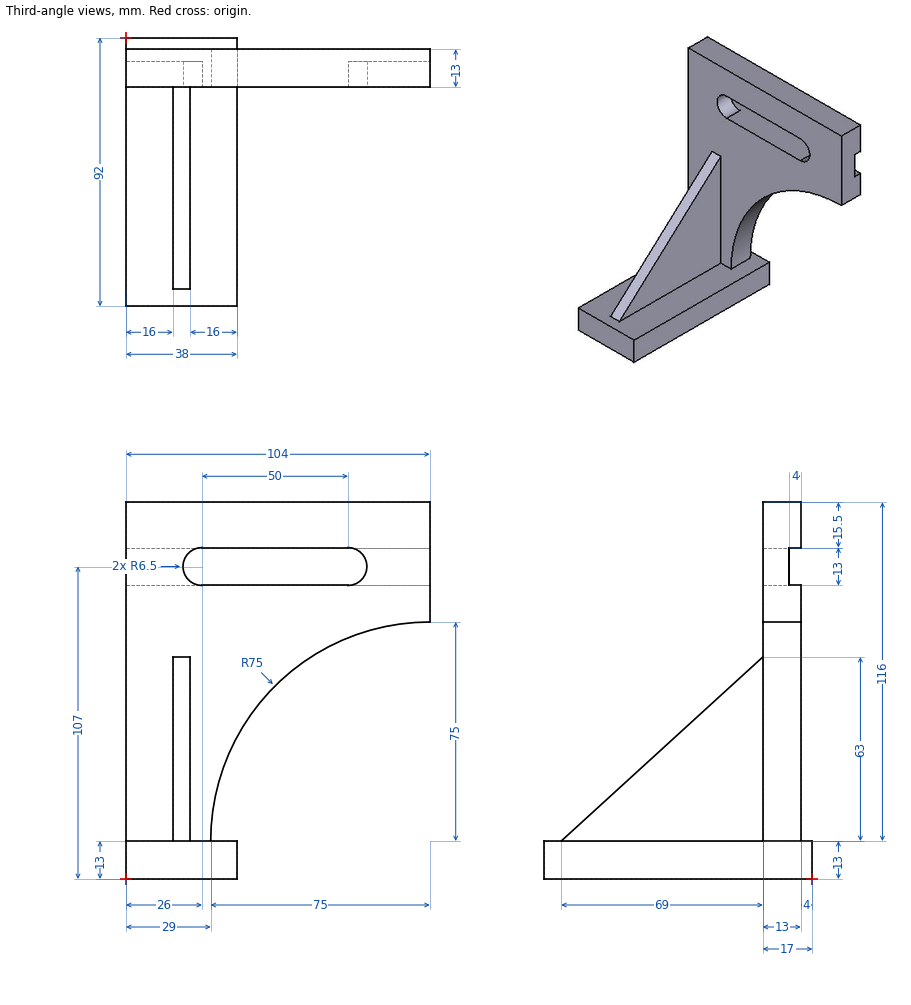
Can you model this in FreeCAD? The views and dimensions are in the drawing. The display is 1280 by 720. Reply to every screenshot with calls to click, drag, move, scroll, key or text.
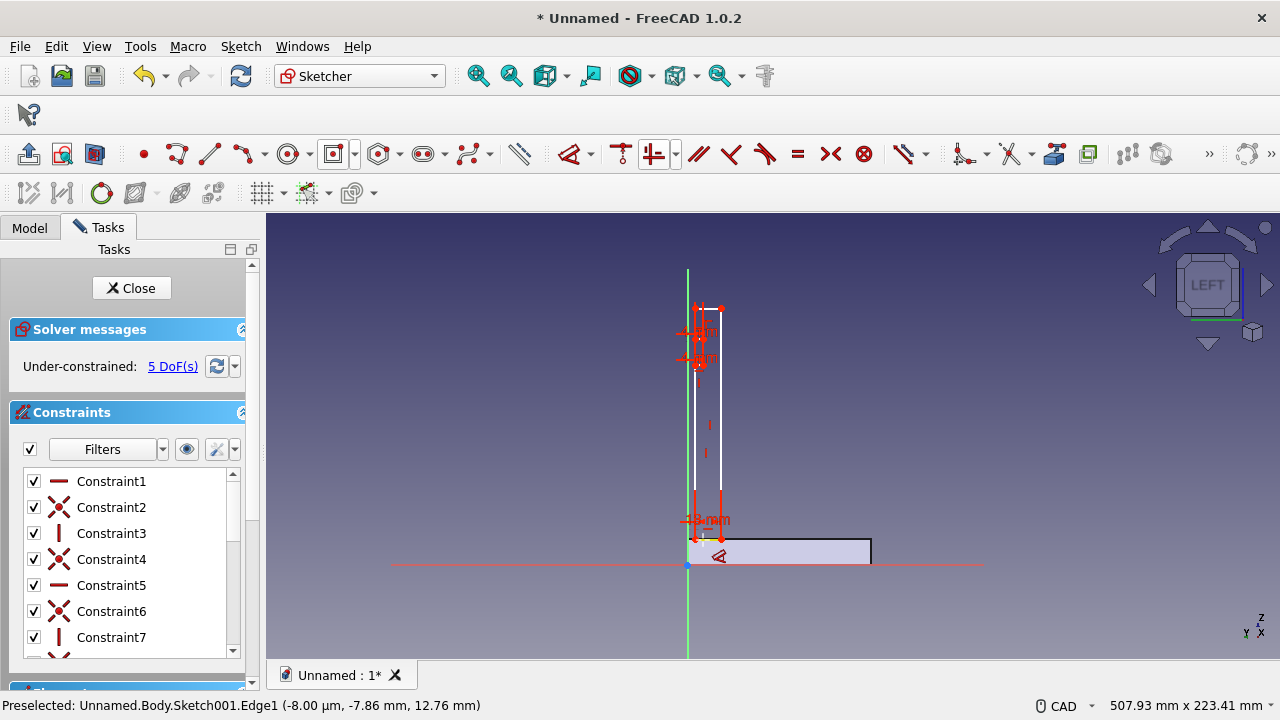
scroll(703, 347, up, 3)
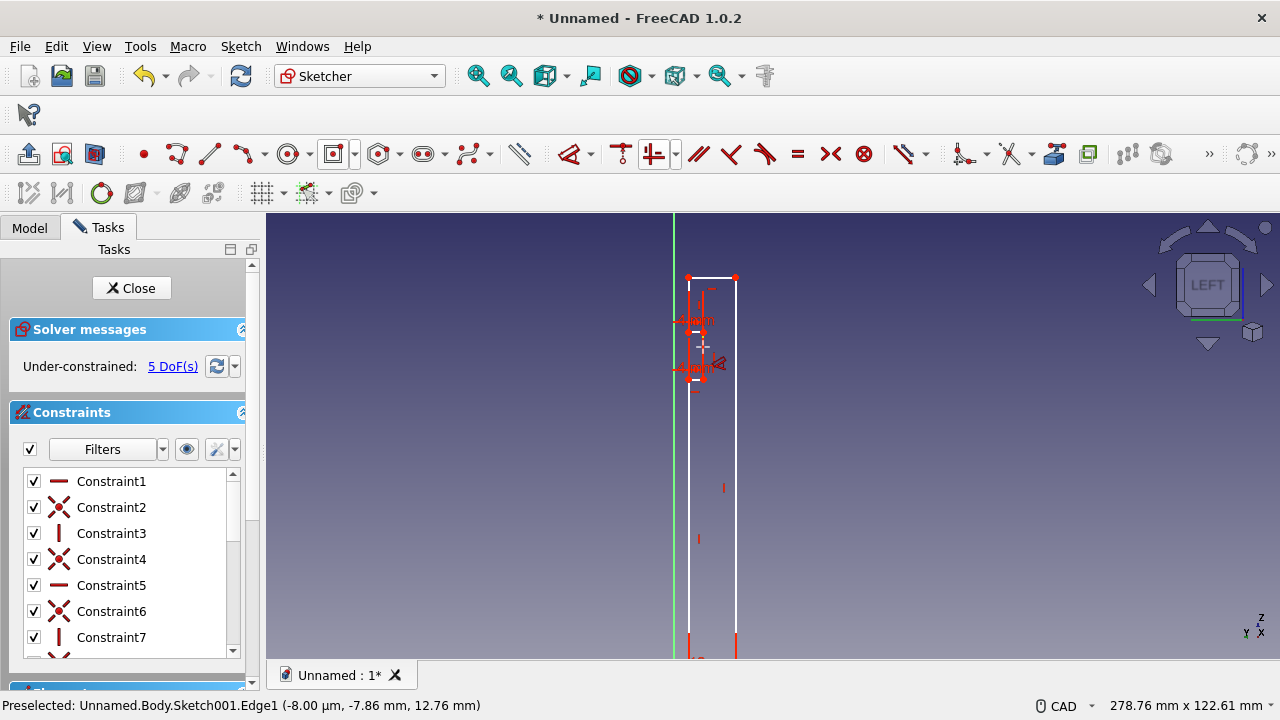
click(703, 347)
click(645, 345)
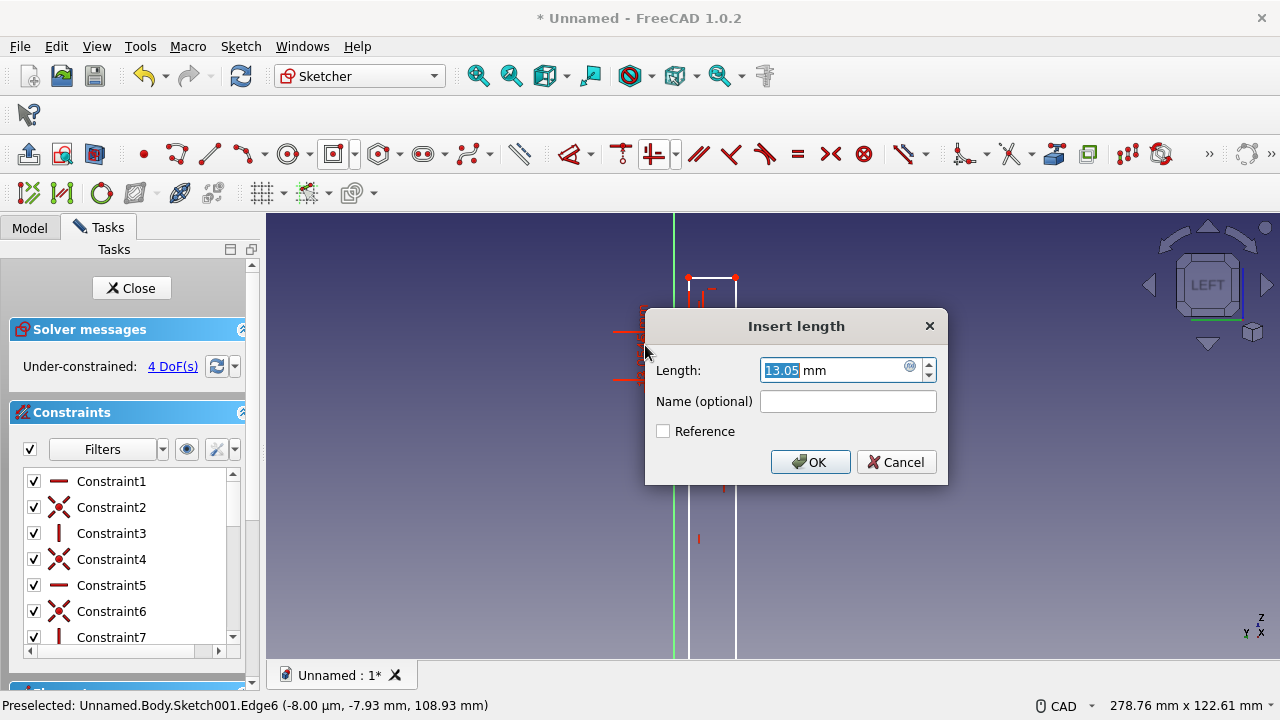
text(13)
key(Return)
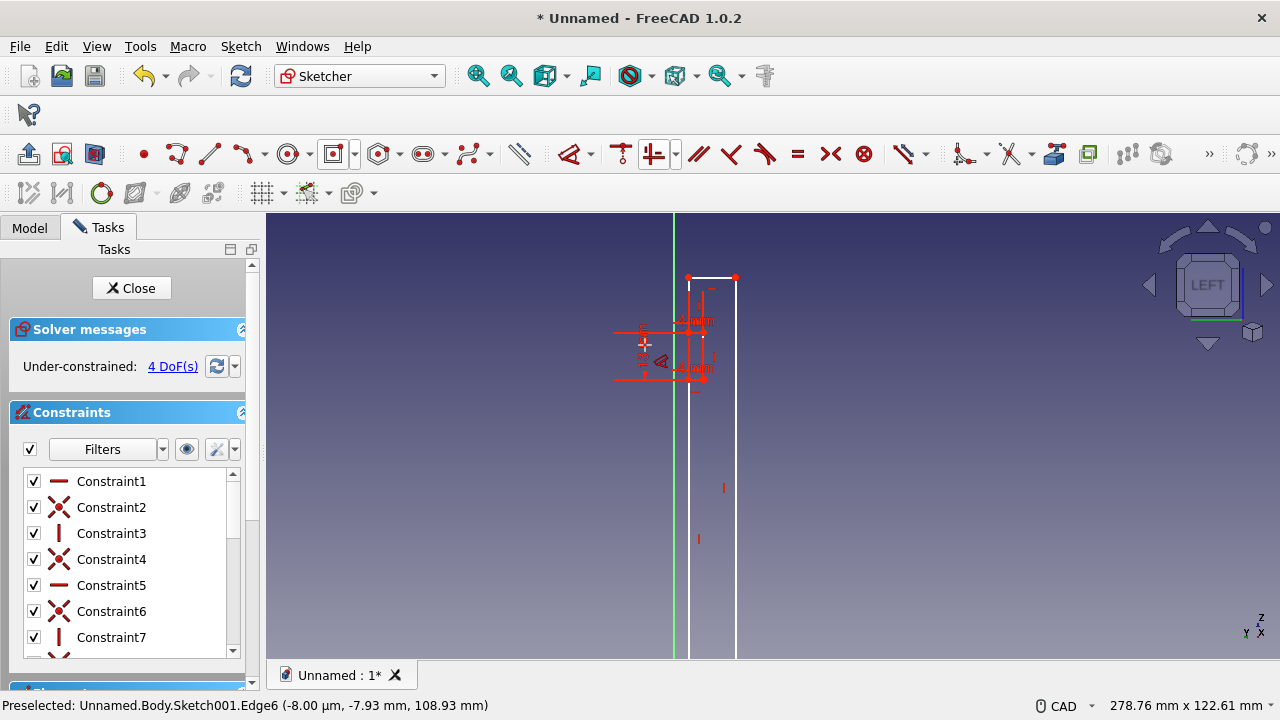
scroll(703, 346, down, 3)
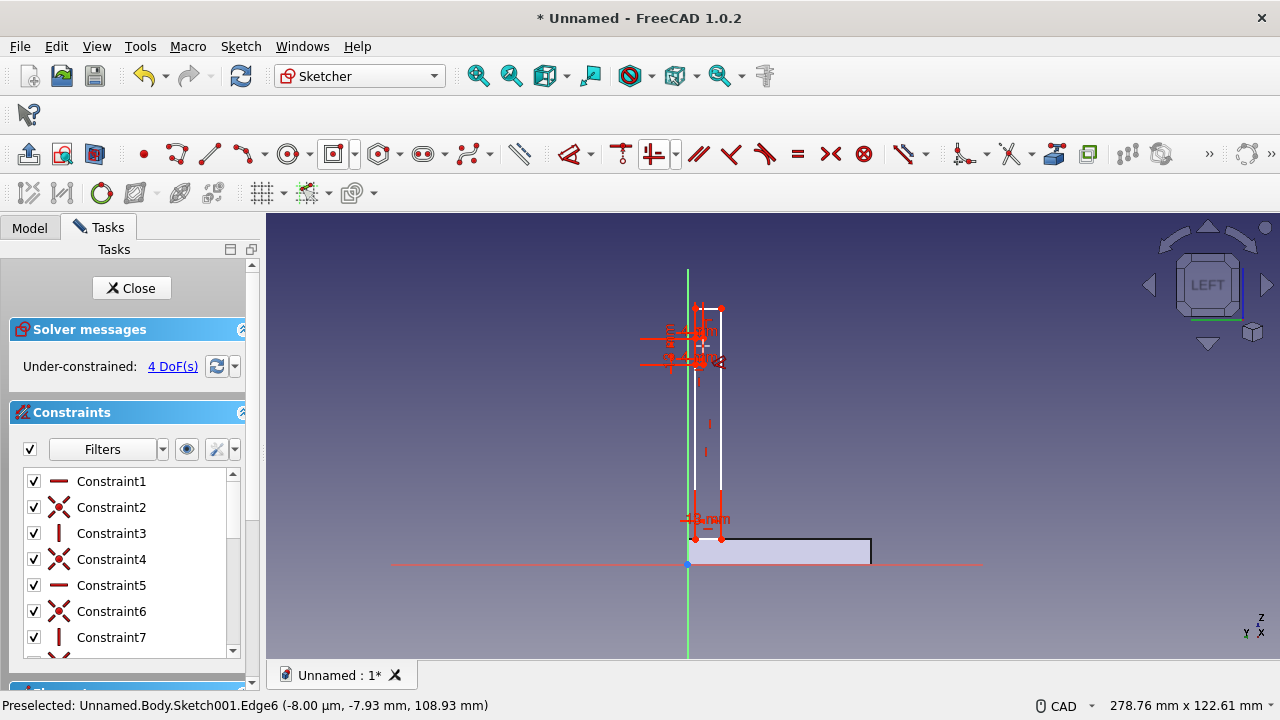
scroll(695, 539, up, 9)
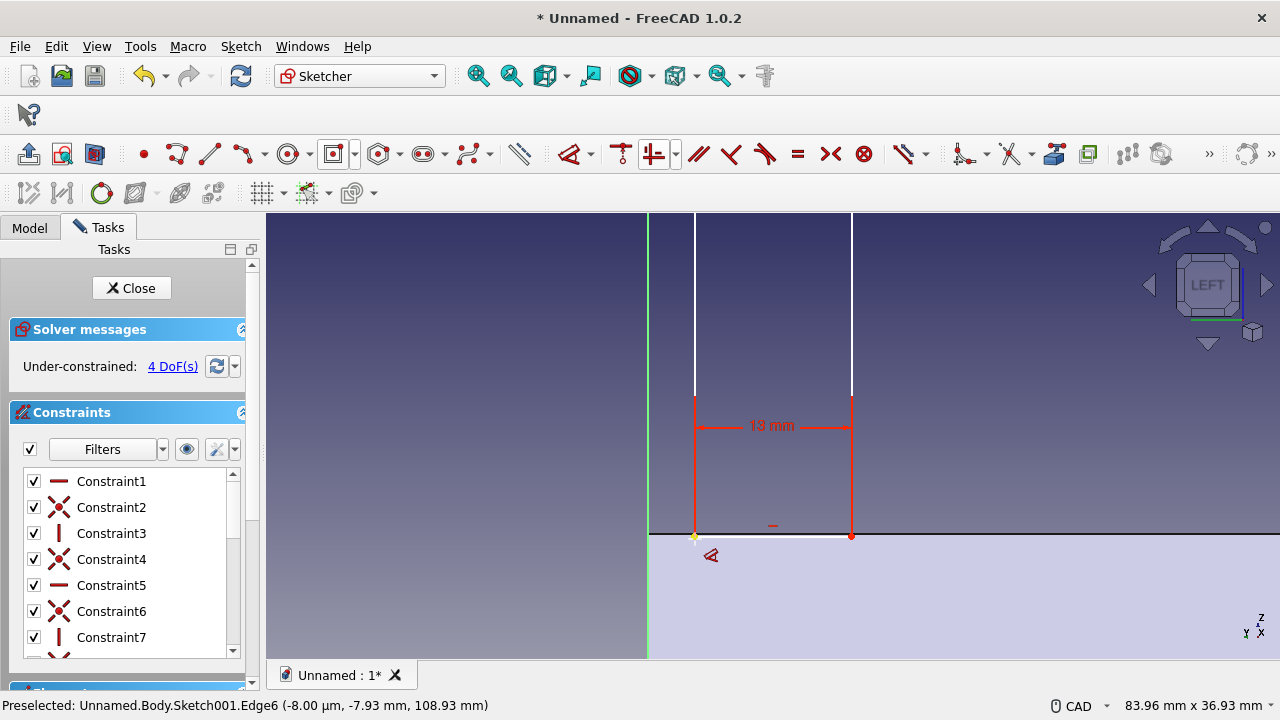
click(695, 537)
click(671, 503)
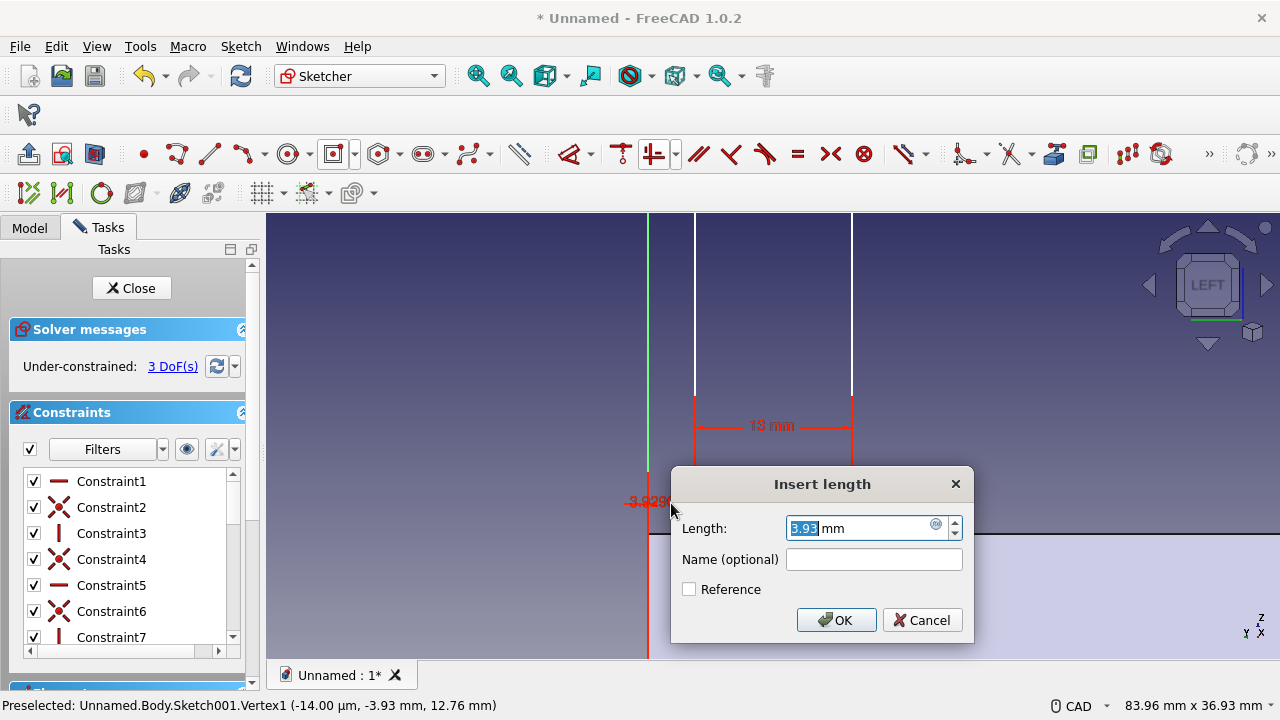
text(4)
key(Return)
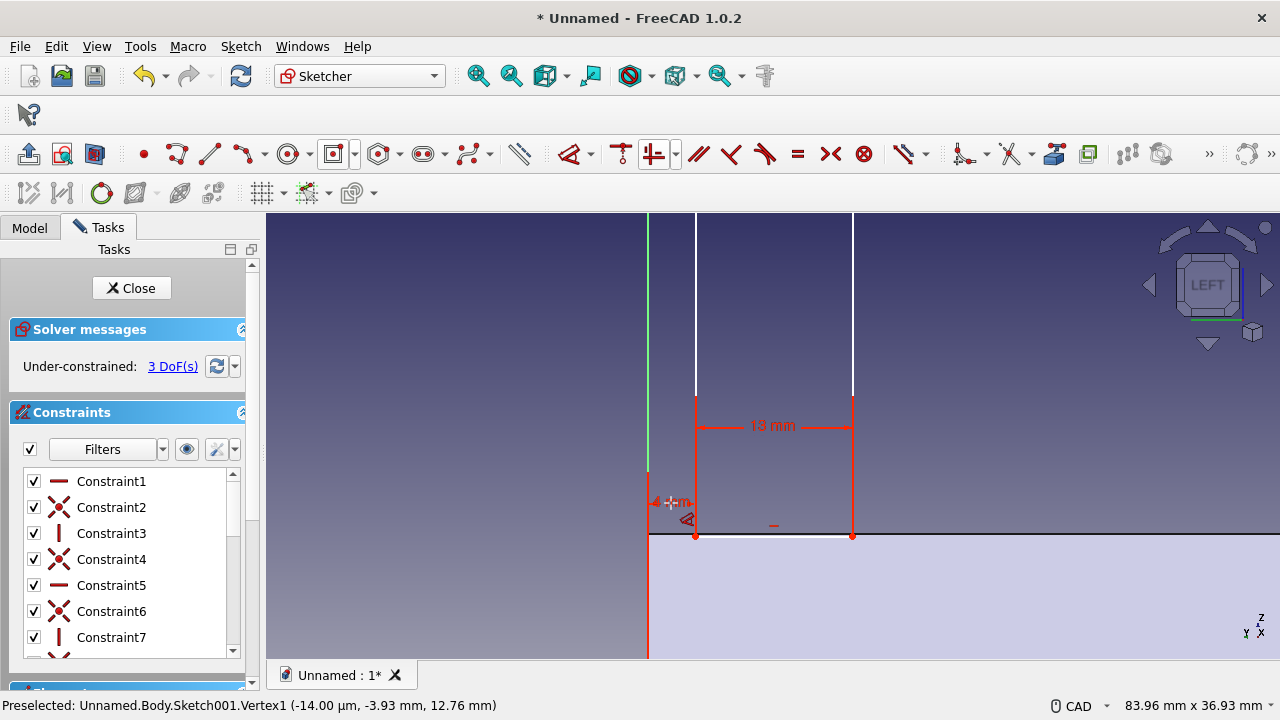
scroll(695, 540, down, 9)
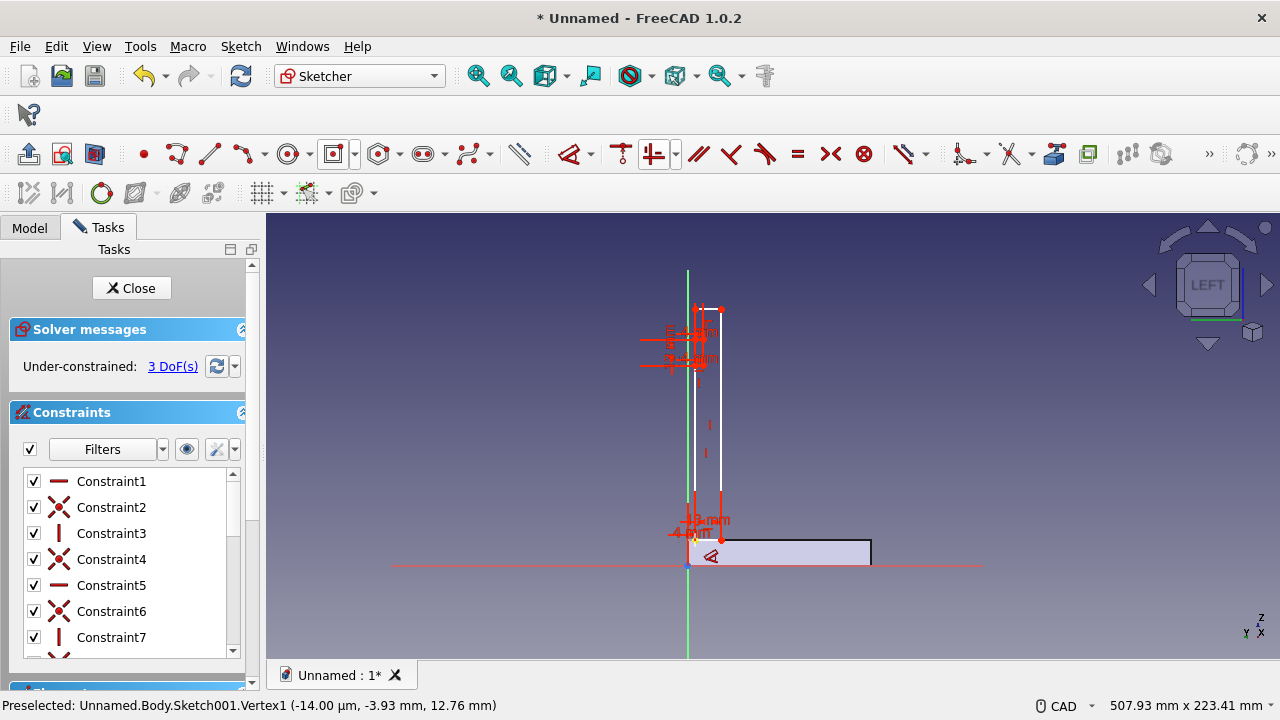
click(721, 494)
click(755, 425)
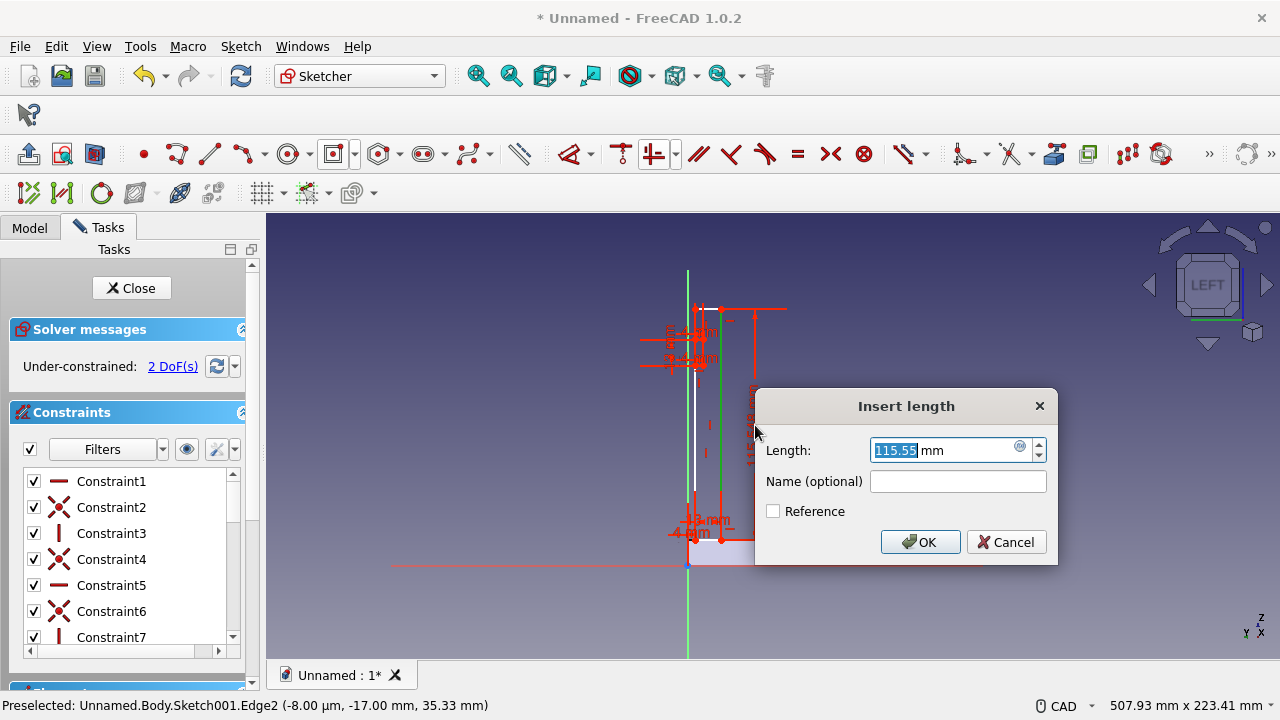
text(116)
key(Return)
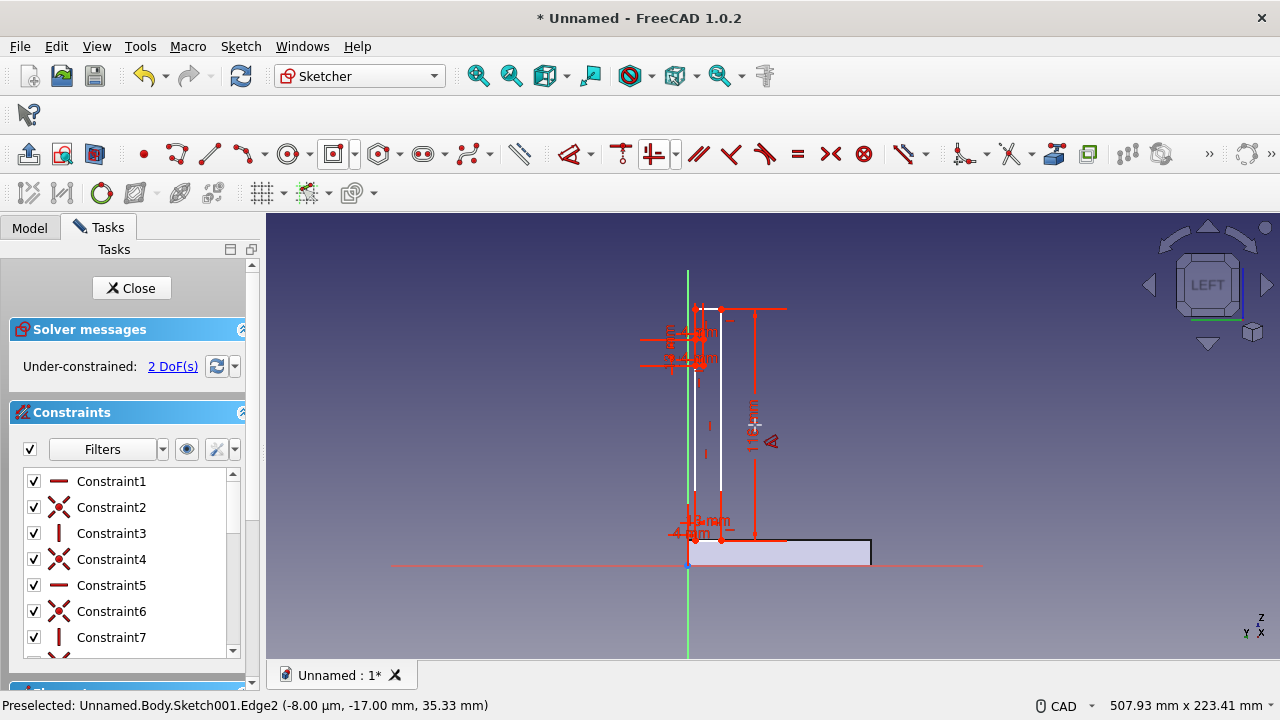
scroll(695, 541, up, 3)